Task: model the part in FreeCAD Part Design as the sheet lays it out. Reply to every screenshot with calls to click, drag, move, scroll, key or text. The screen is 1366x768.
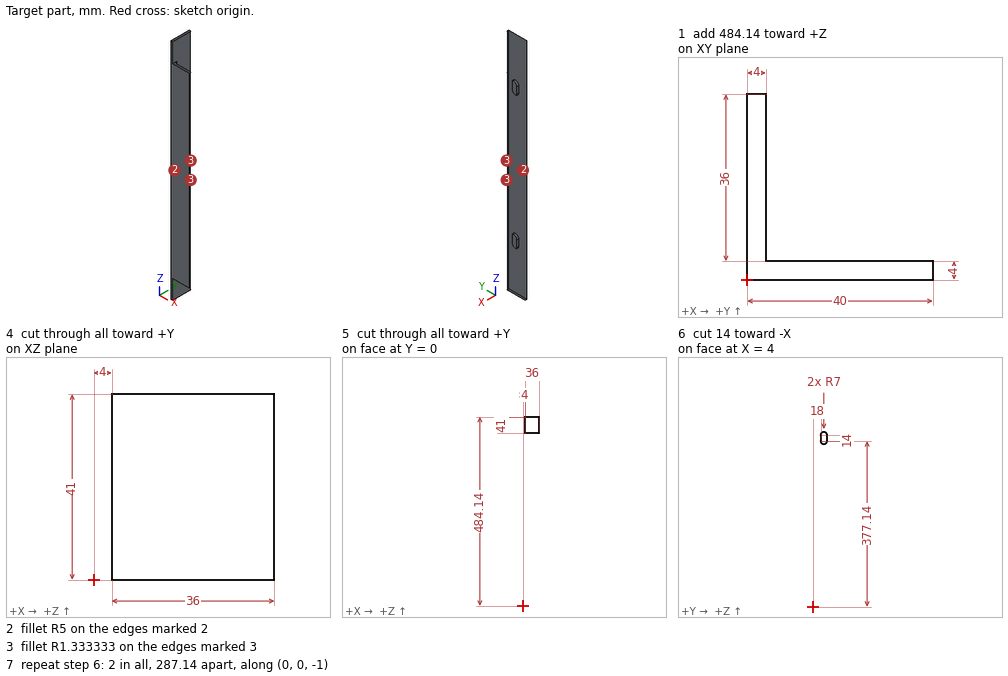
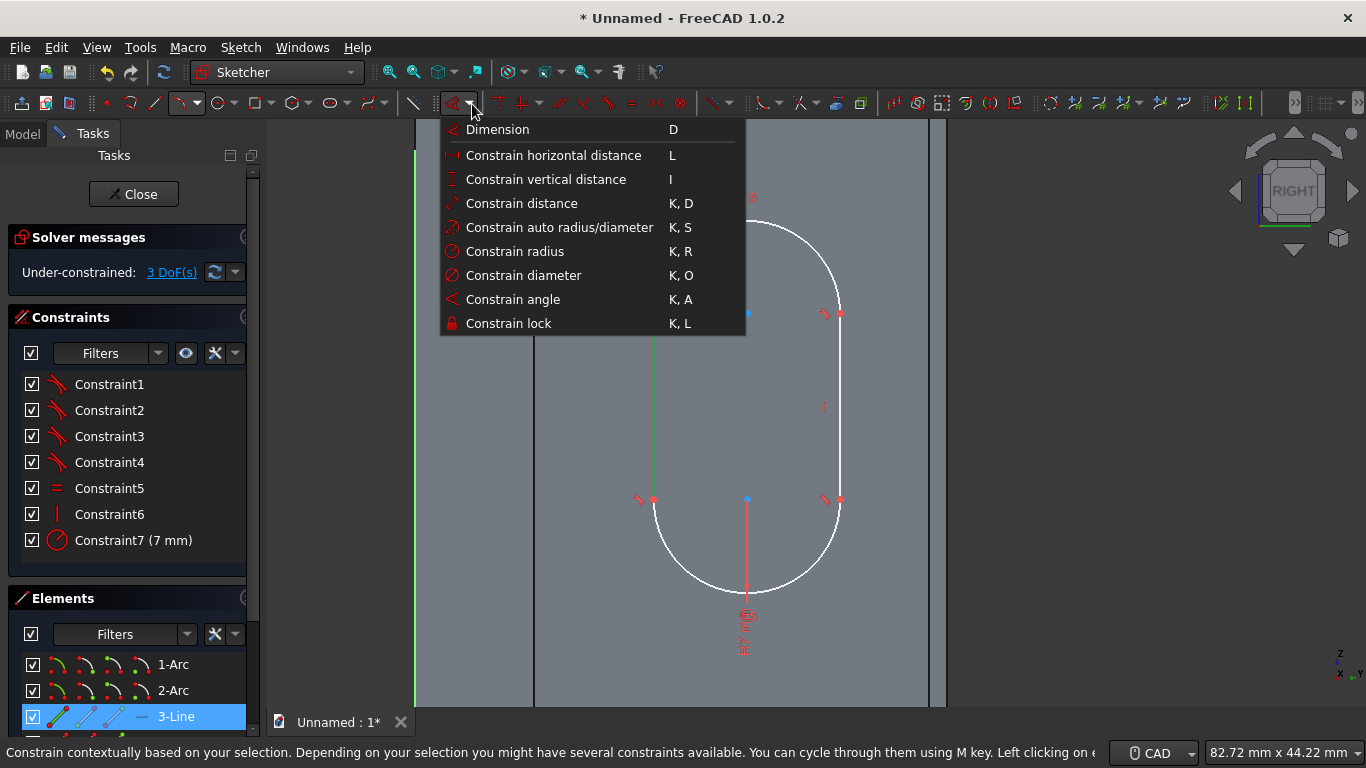
click(593, 179)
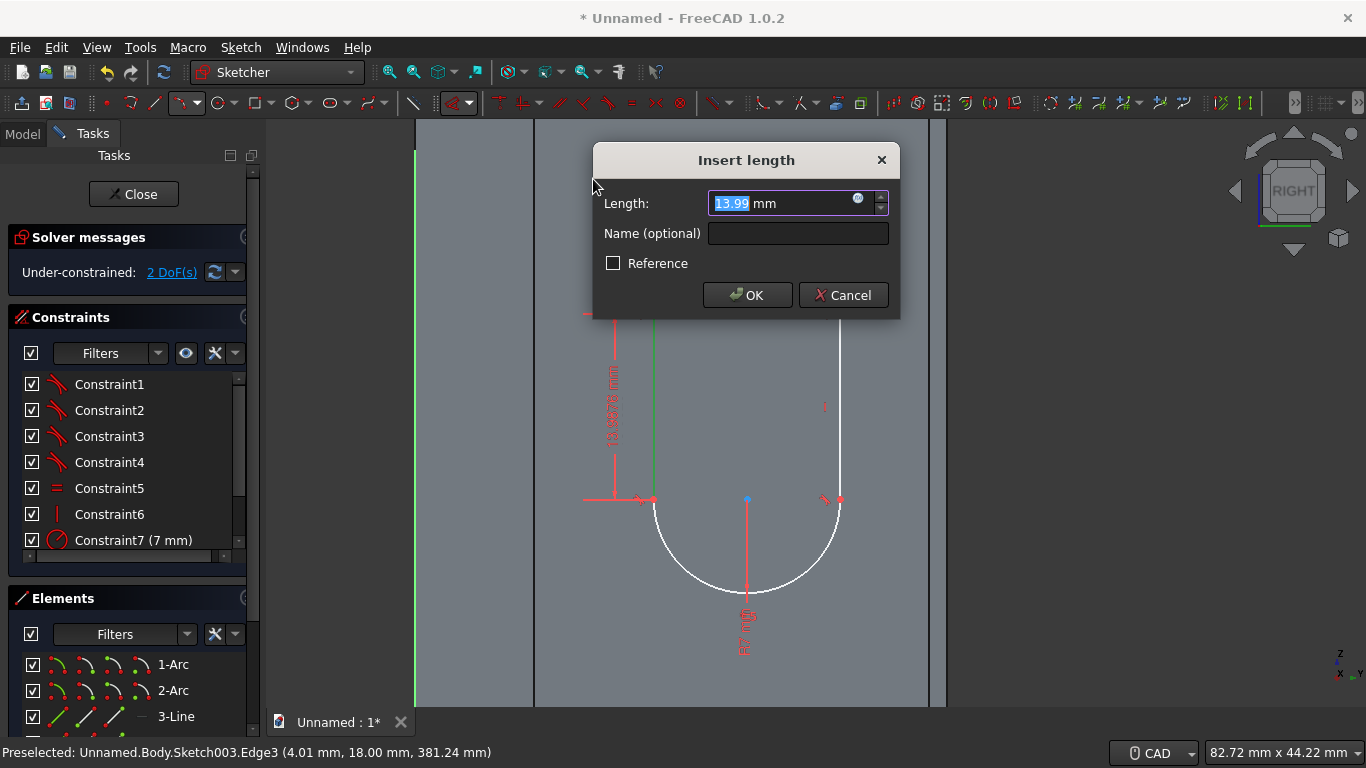
text(14)
key(Return)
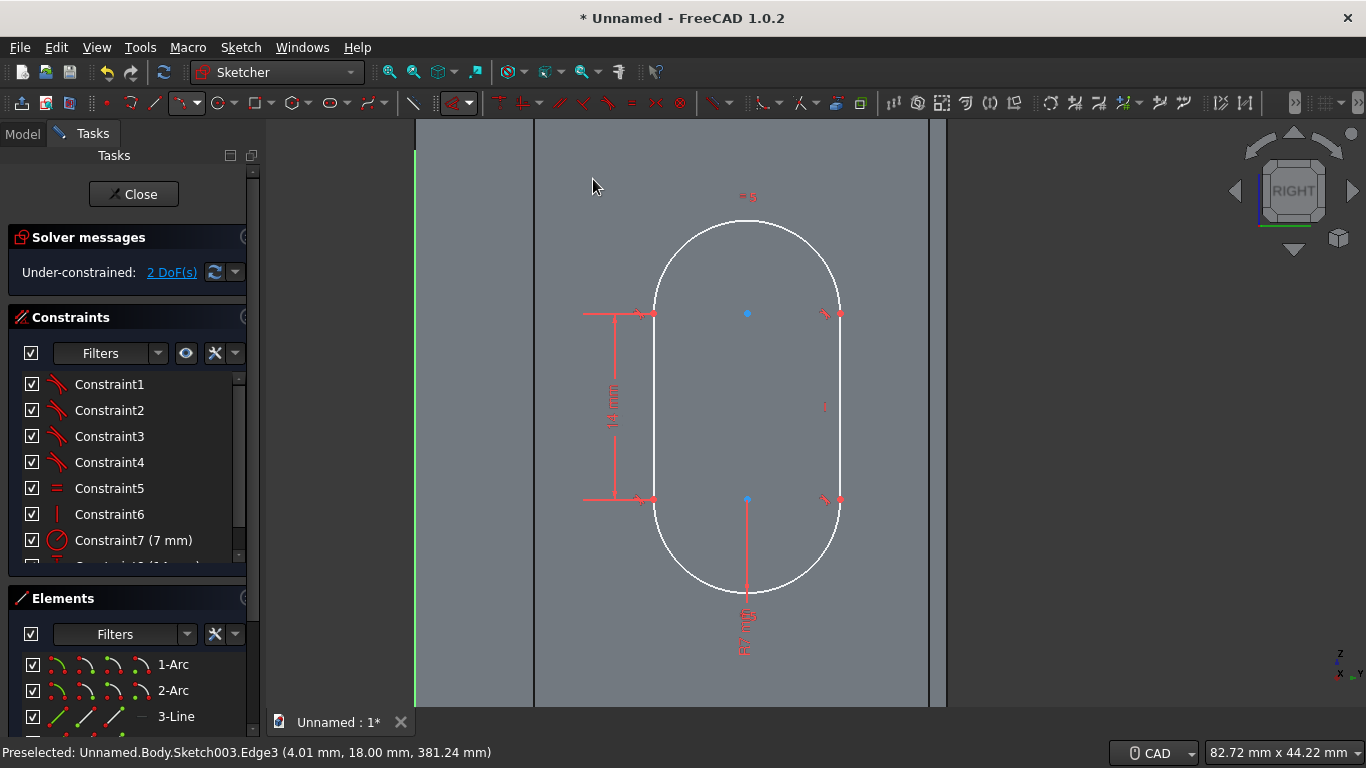
click(654, 500)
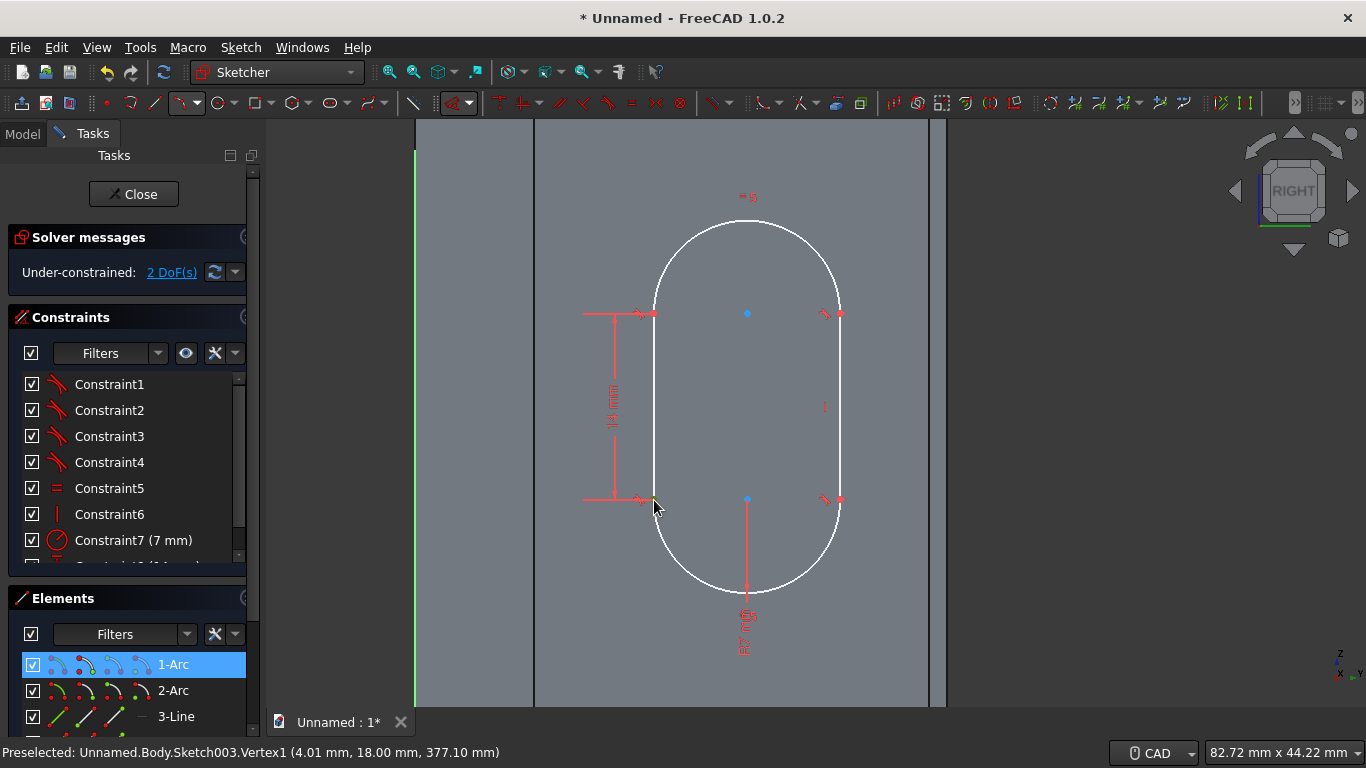
key(l)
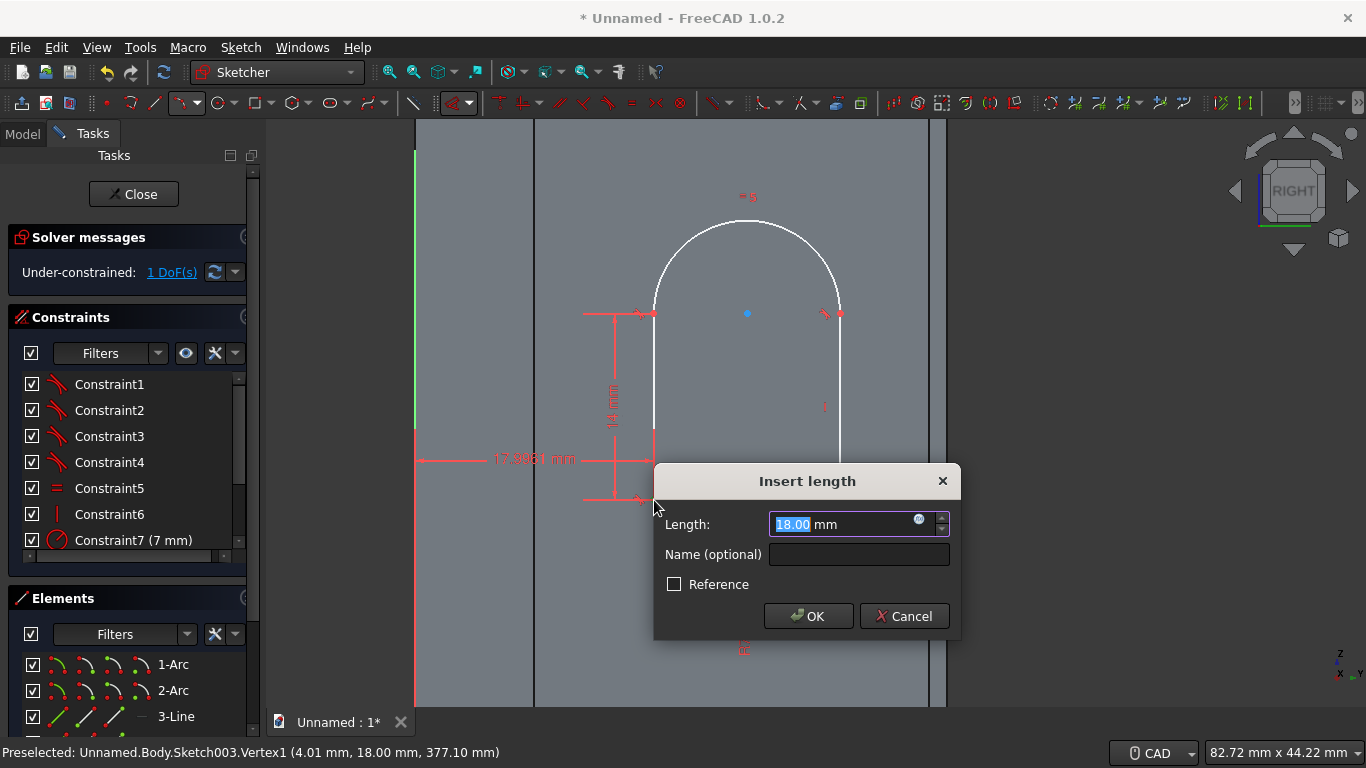
text(18)
key(Return)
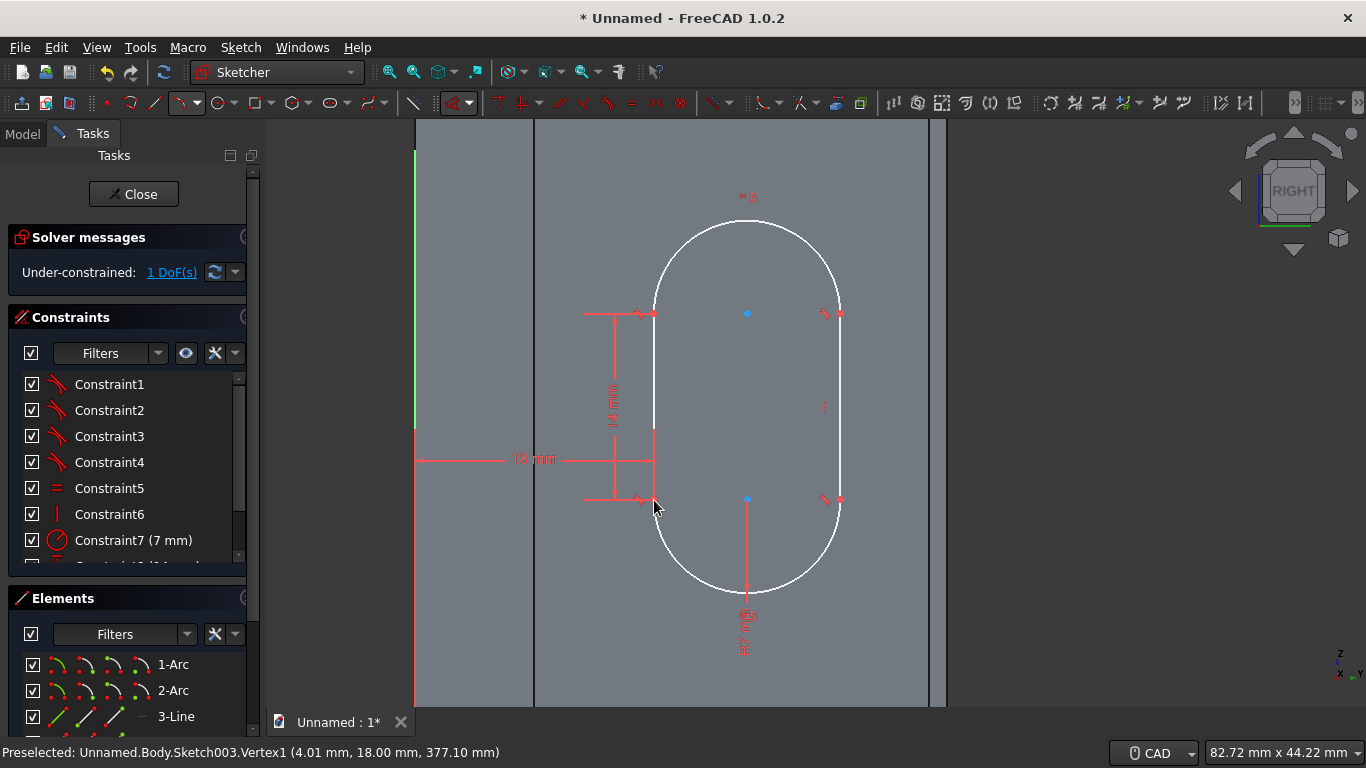
click(654, 500)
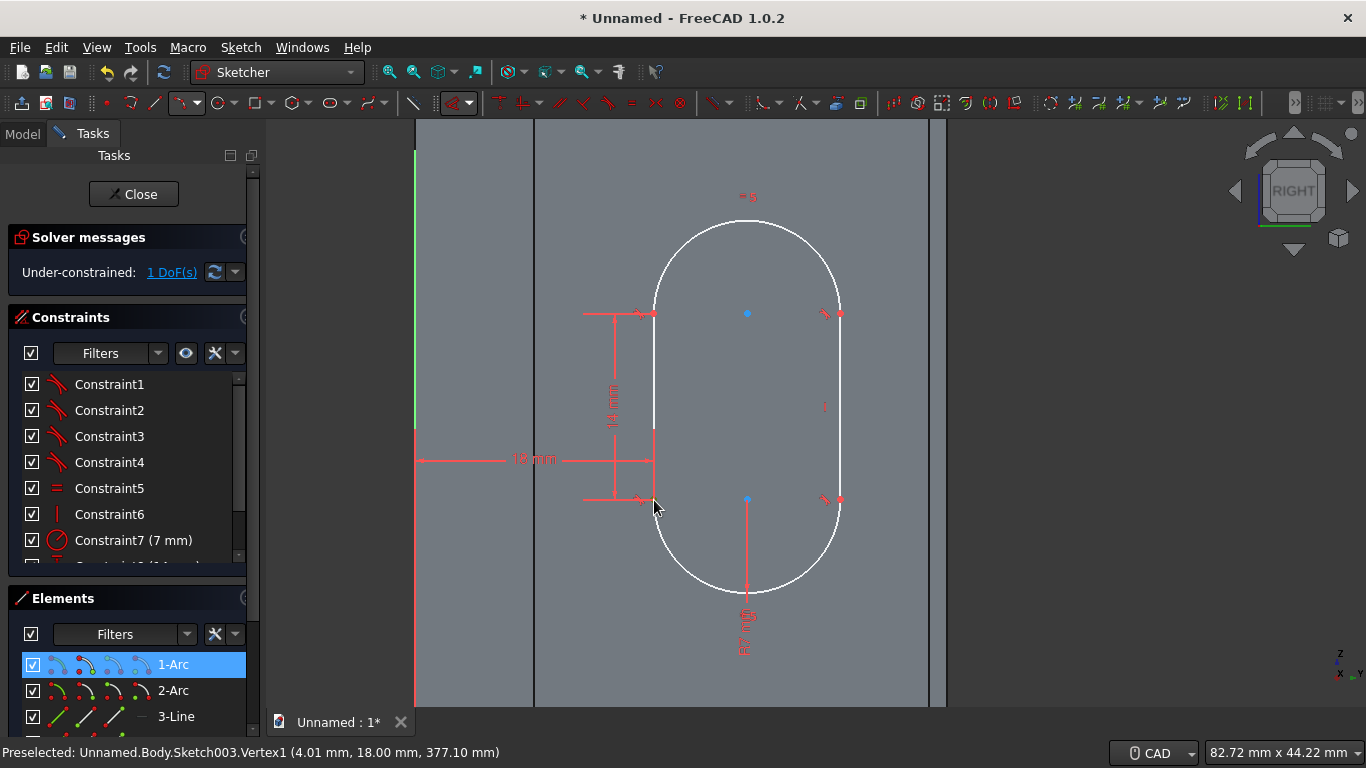
click(472, 104)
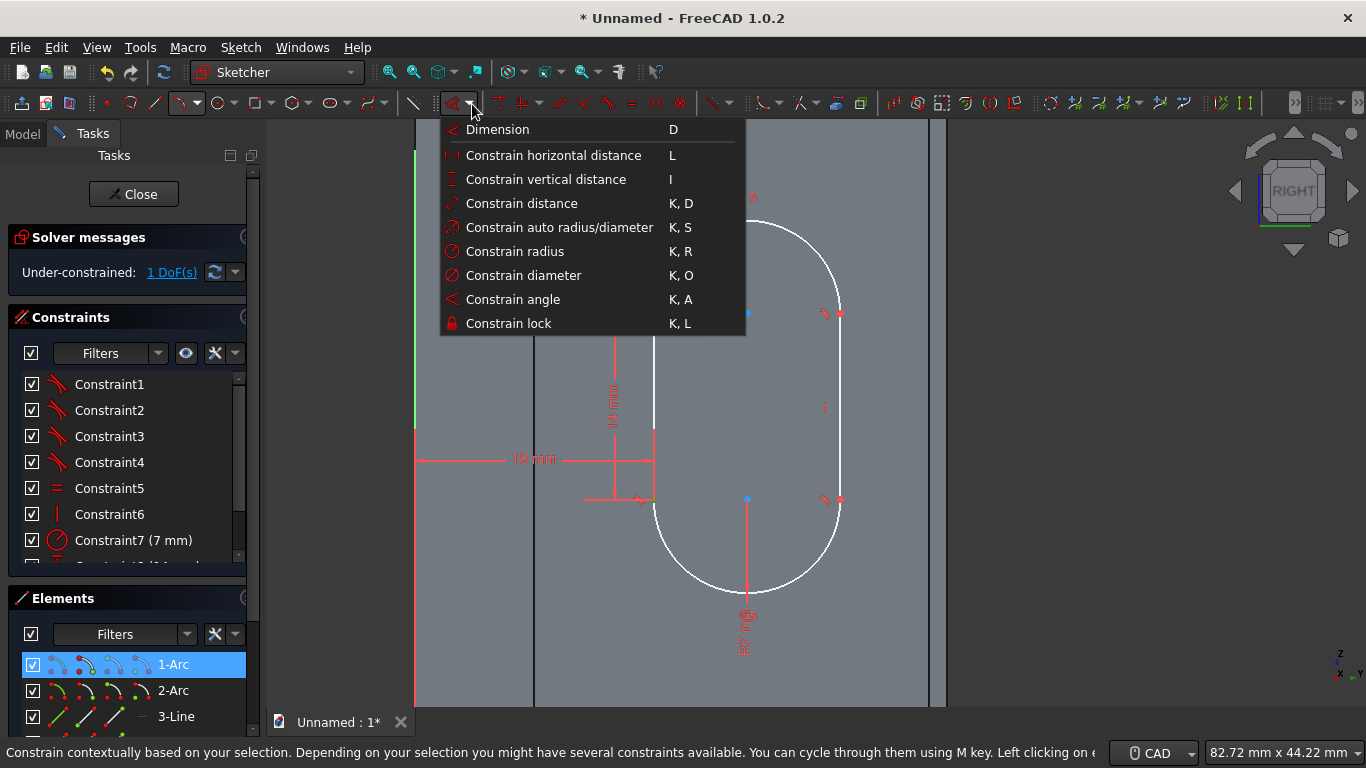
click(593, 179)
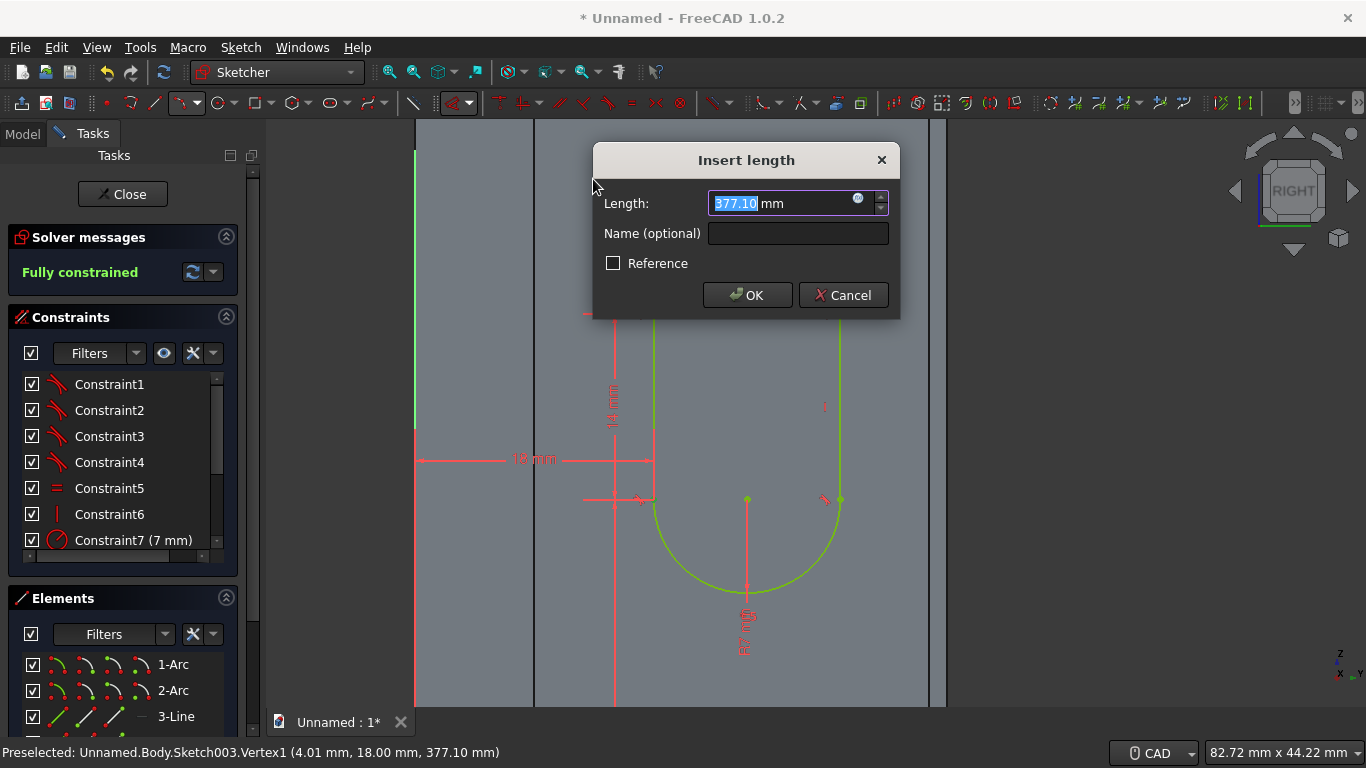
text(377.14)
key(Return)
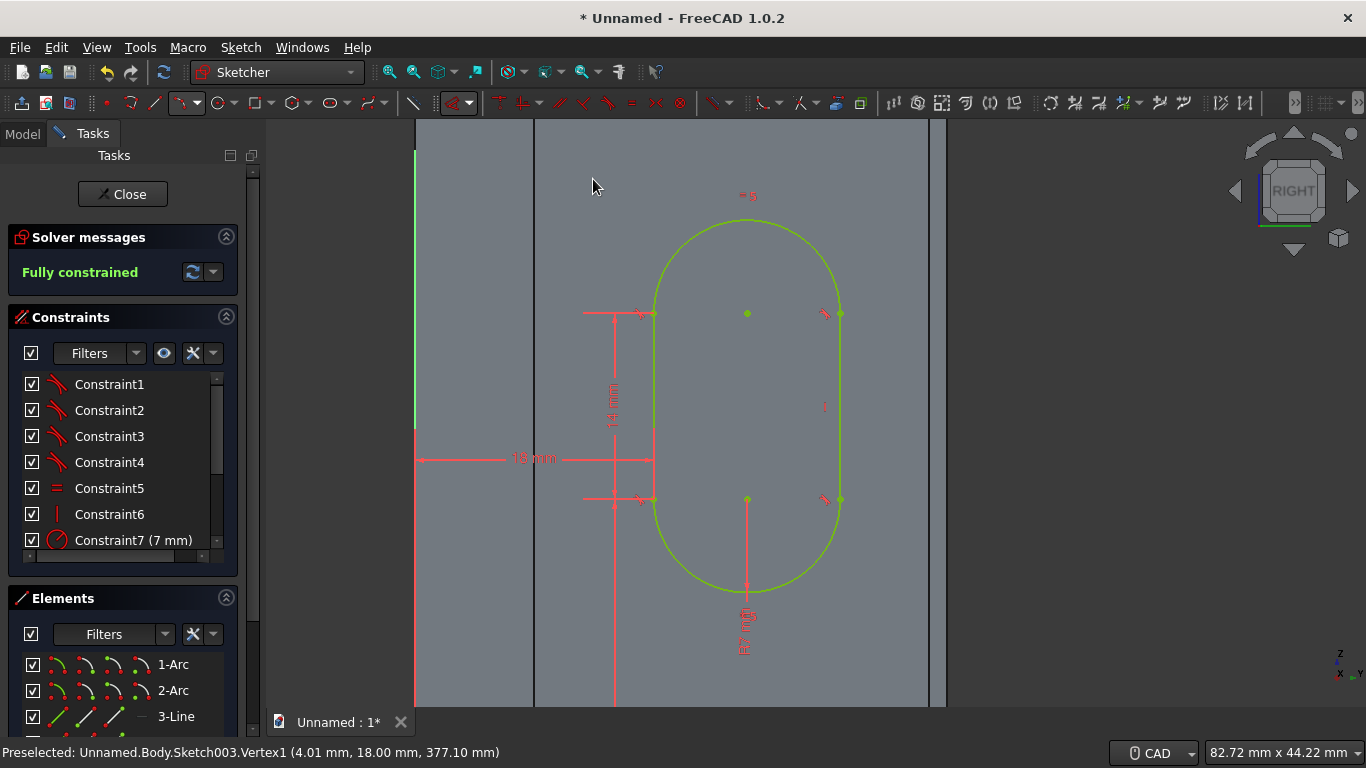
click(123, 194)